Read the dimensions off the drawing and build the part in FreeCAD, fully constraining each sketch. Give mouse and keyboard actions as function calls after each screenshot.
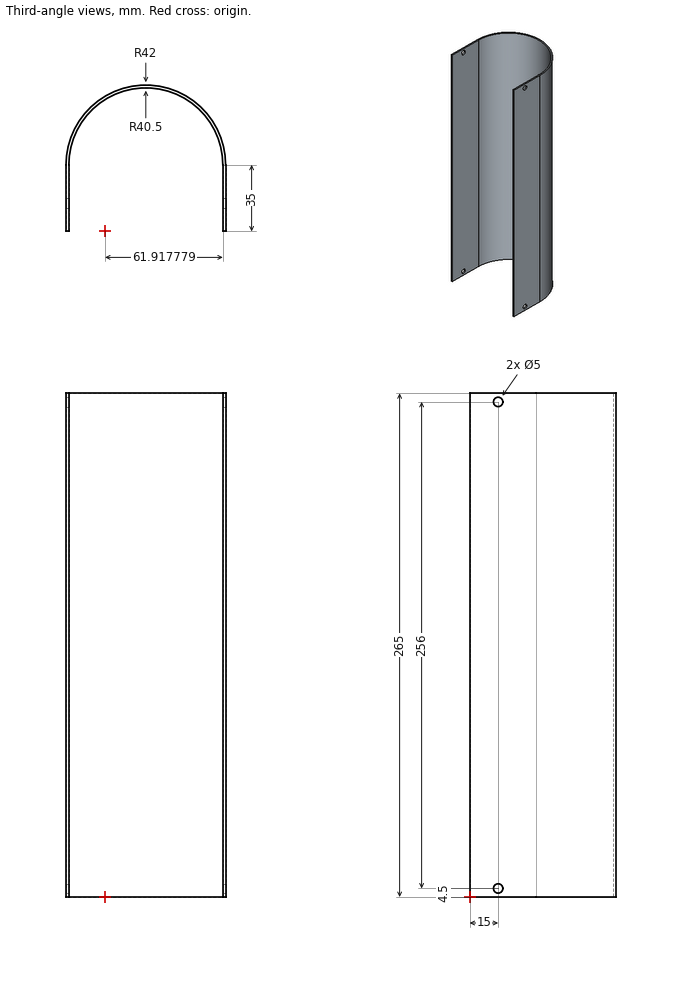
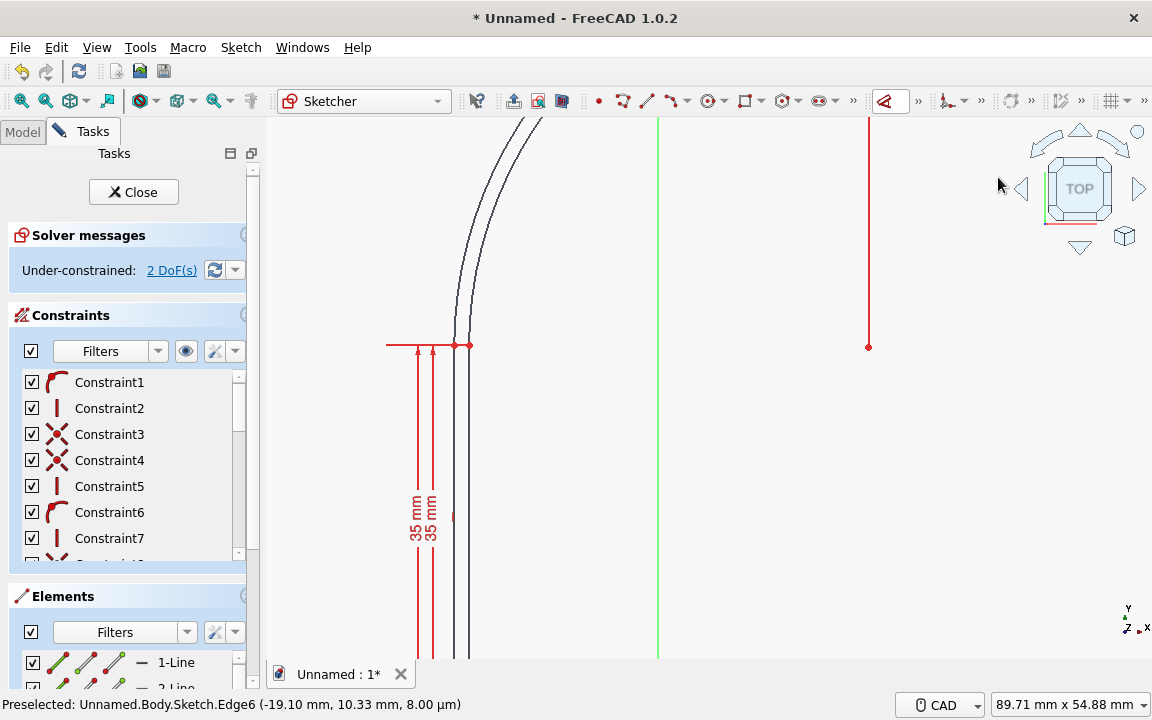
click(869, 347)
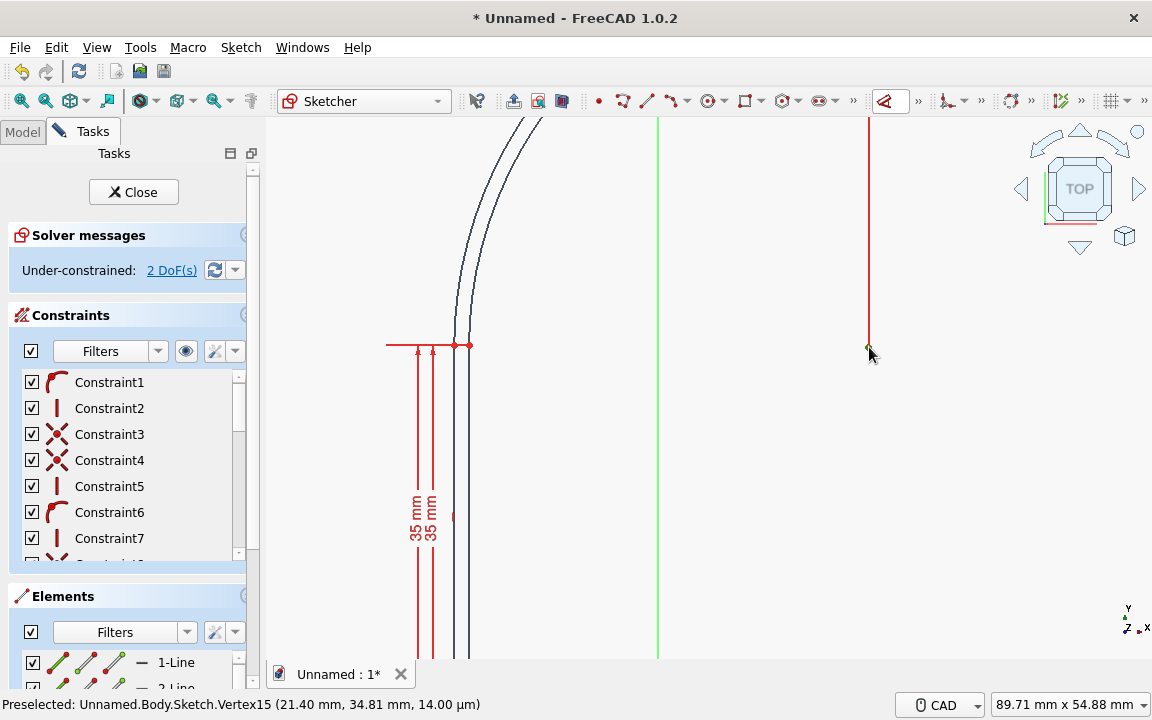
key(i)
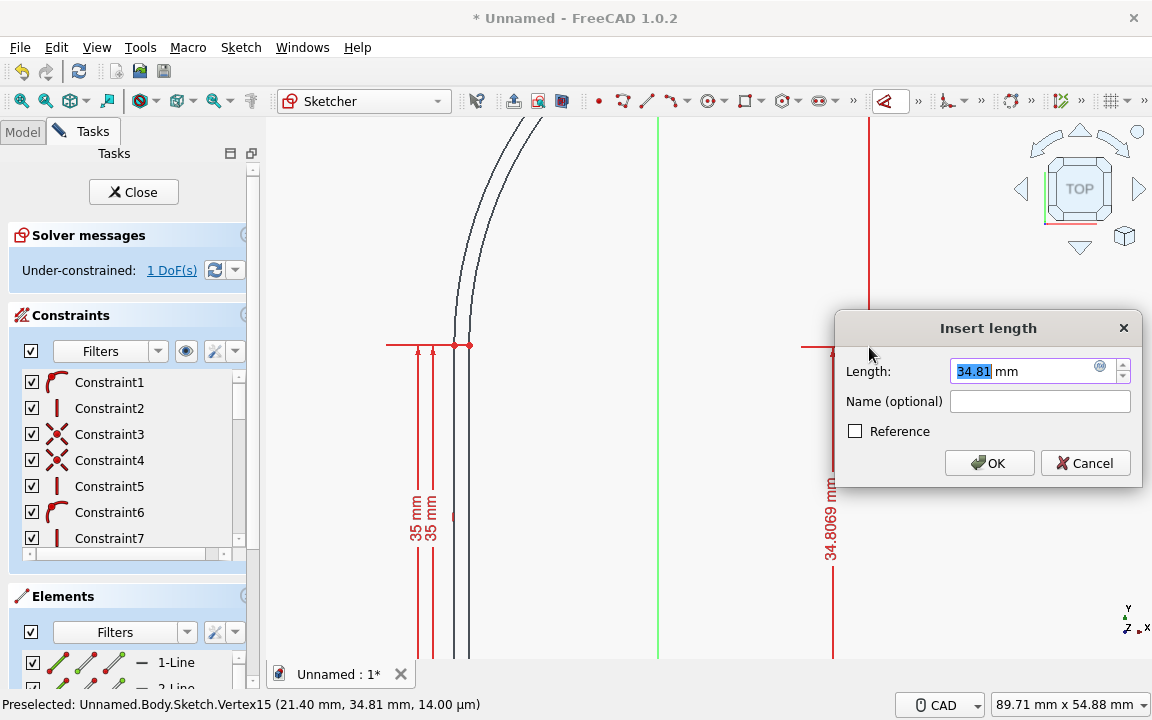
text(35)
key(Return)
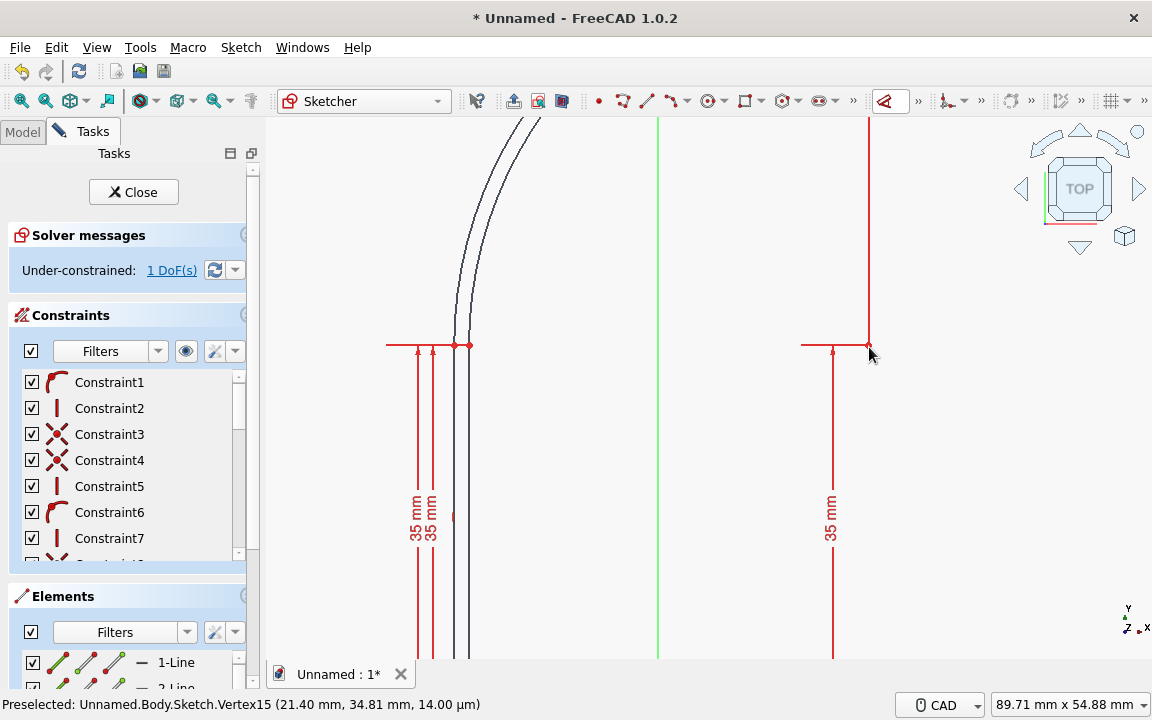
scroll(454, 451, down, 4)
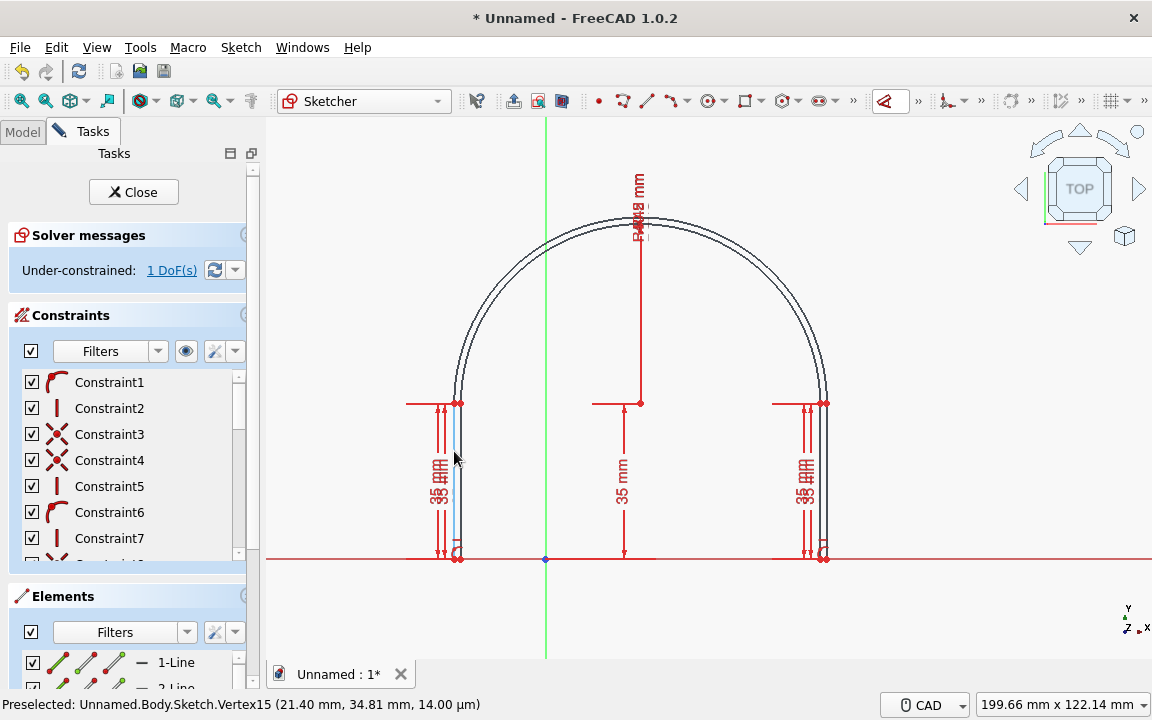
scroll(820, 404, up, 4)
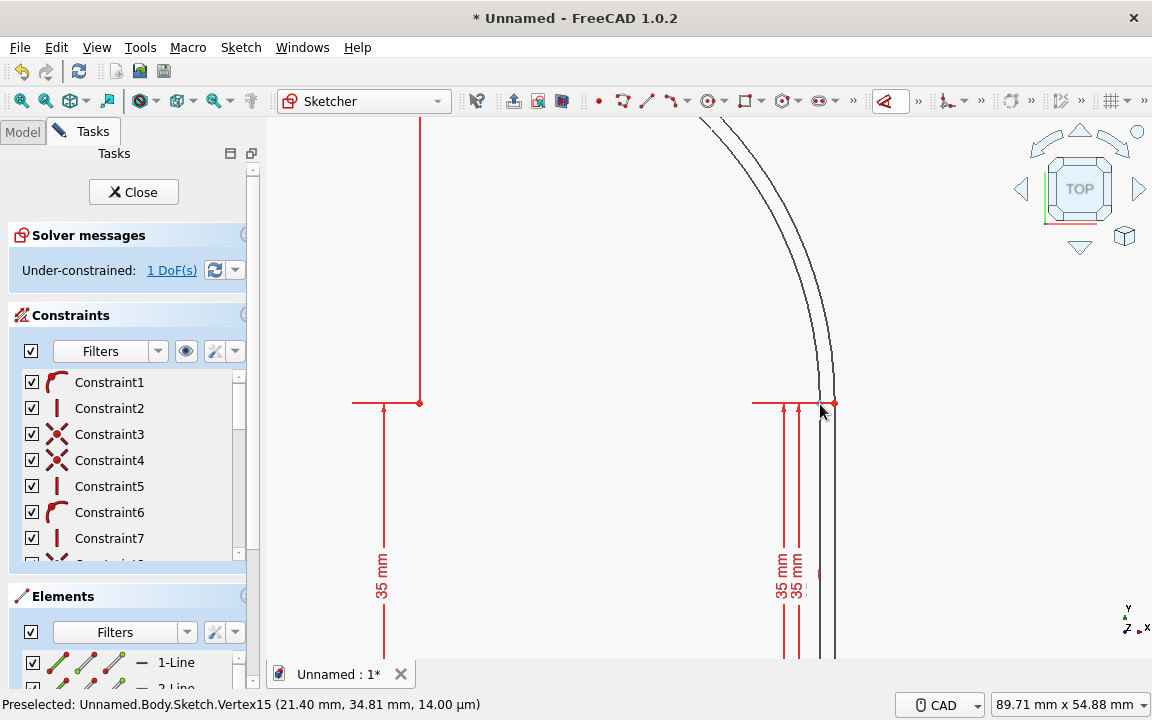
click(820, 403)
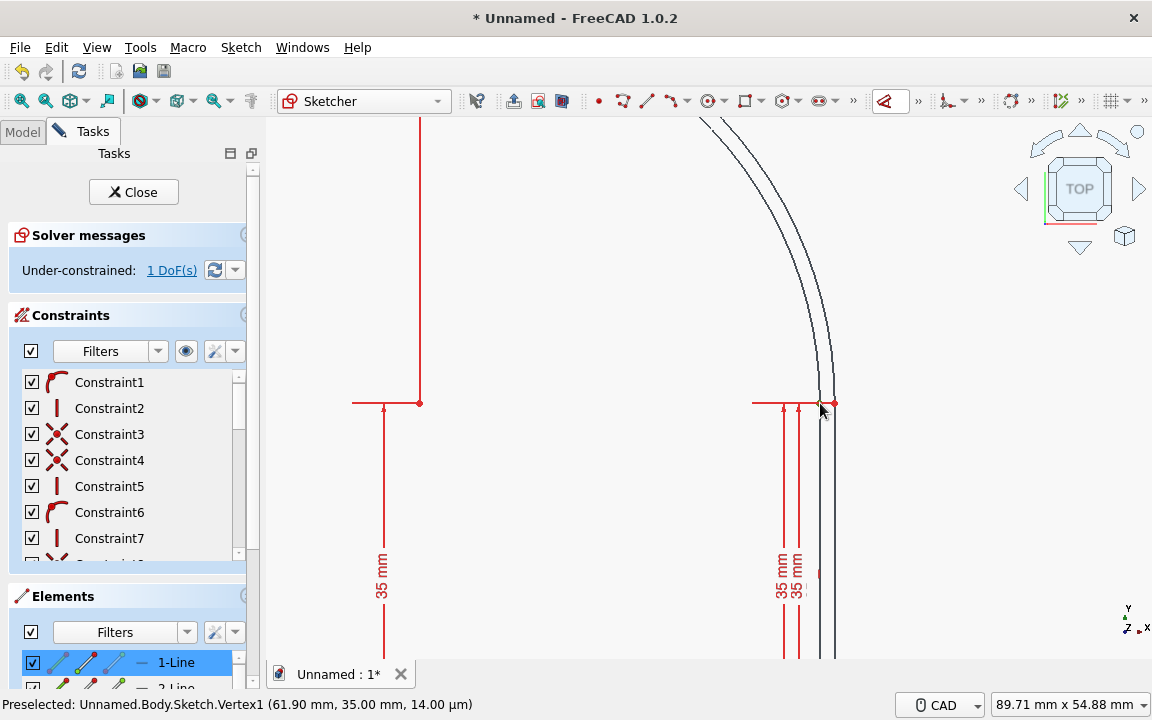
click(904, 102)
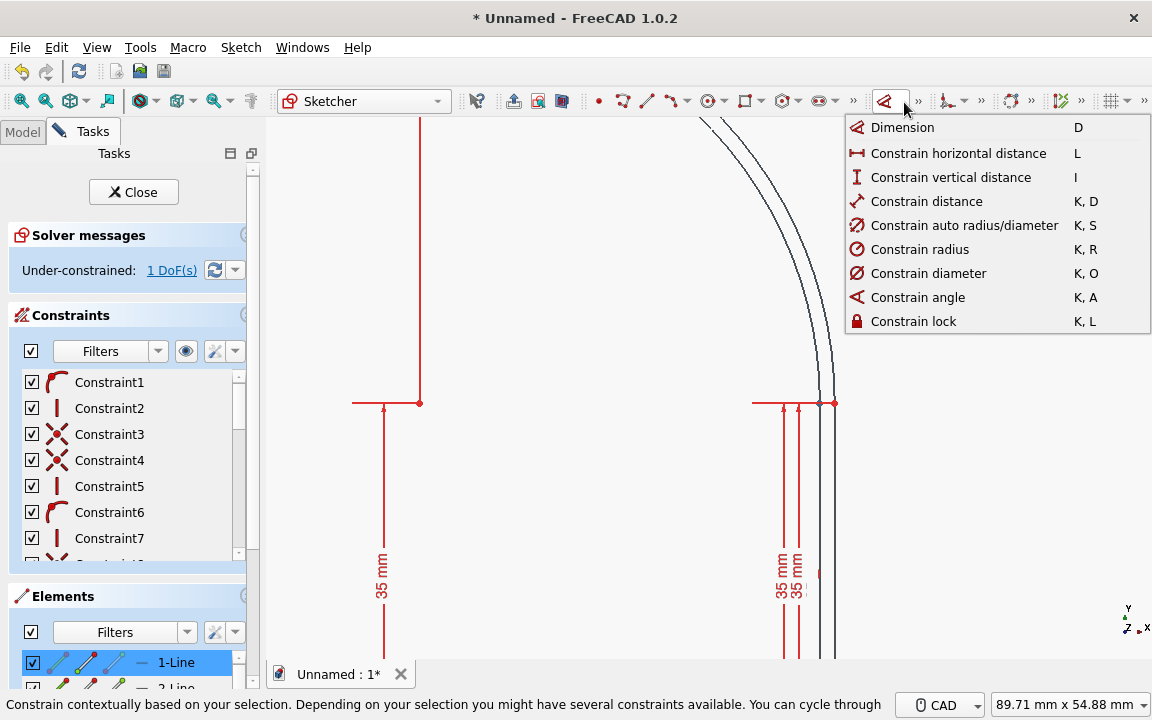
click(998, 153)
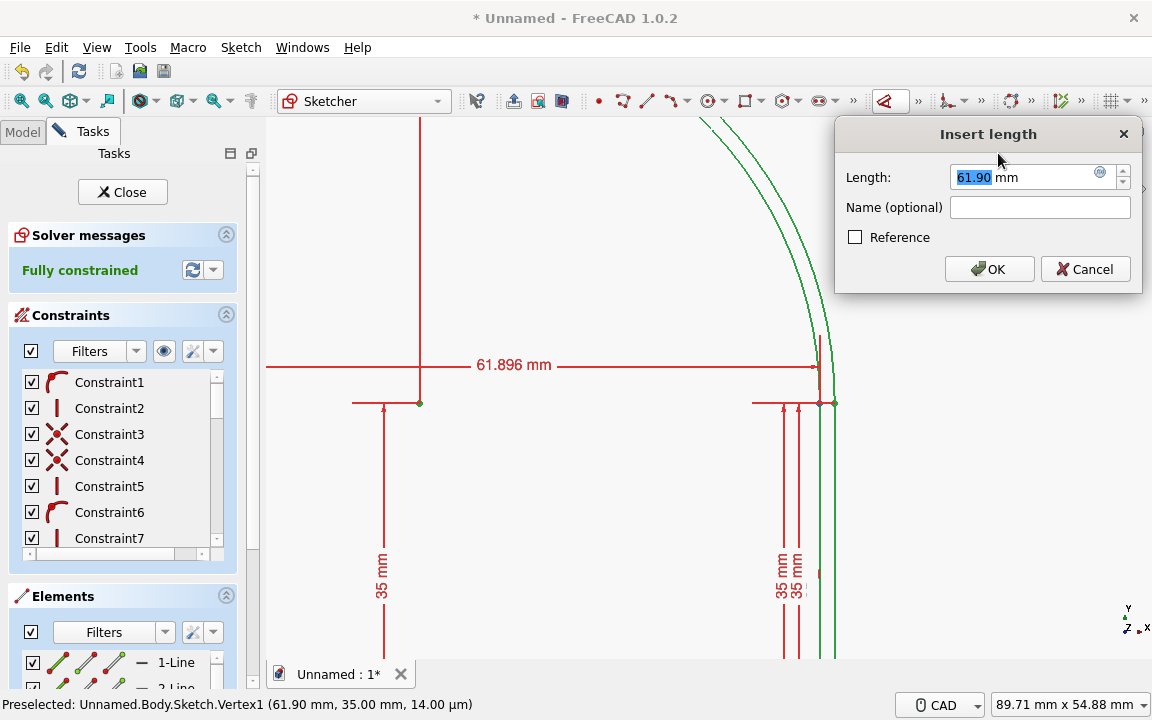
text(61.917779)
key(Return)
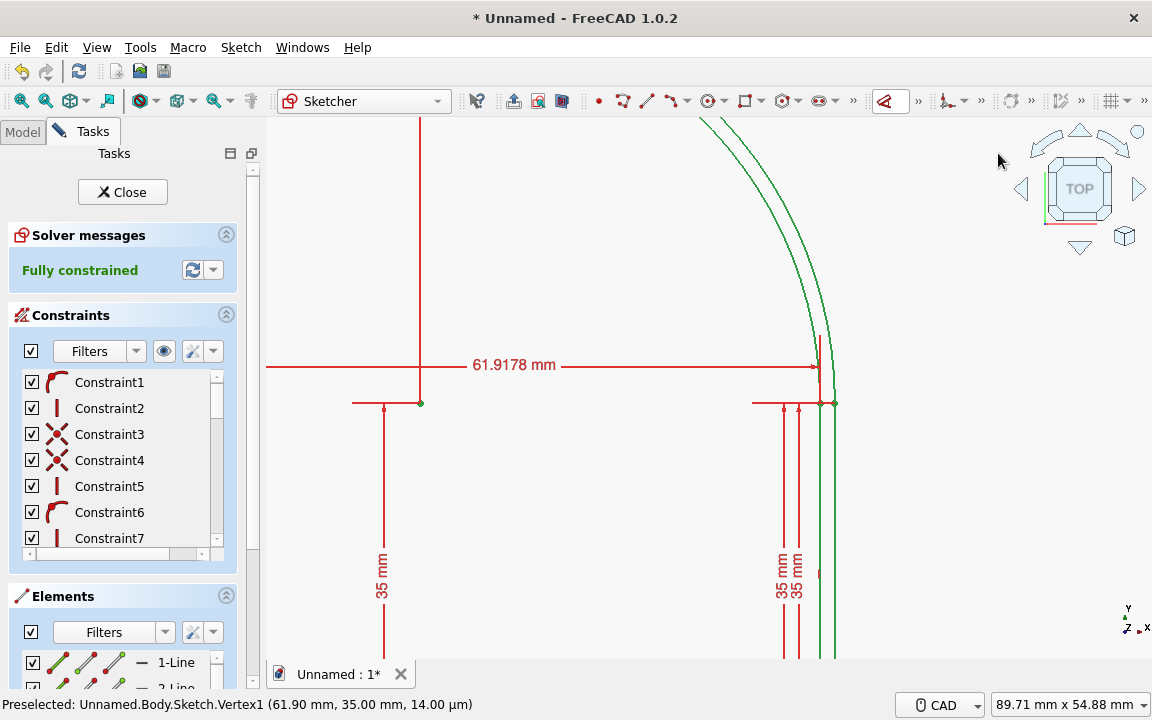
click(123, 192)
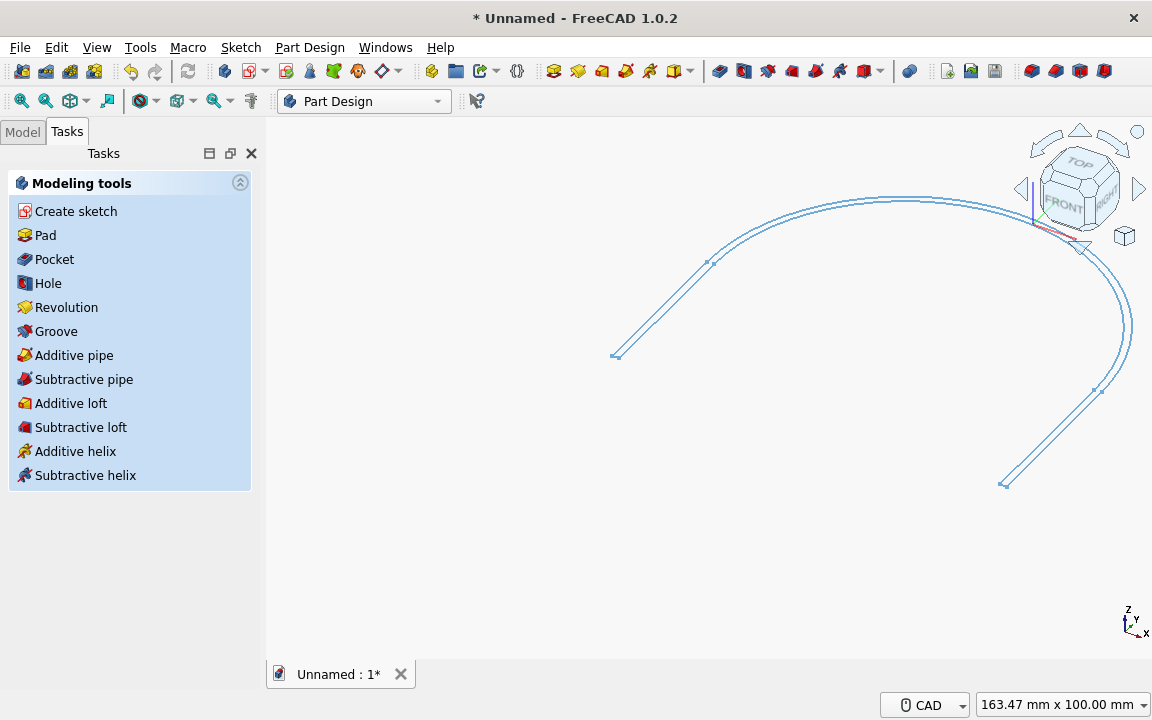
click(554, 72)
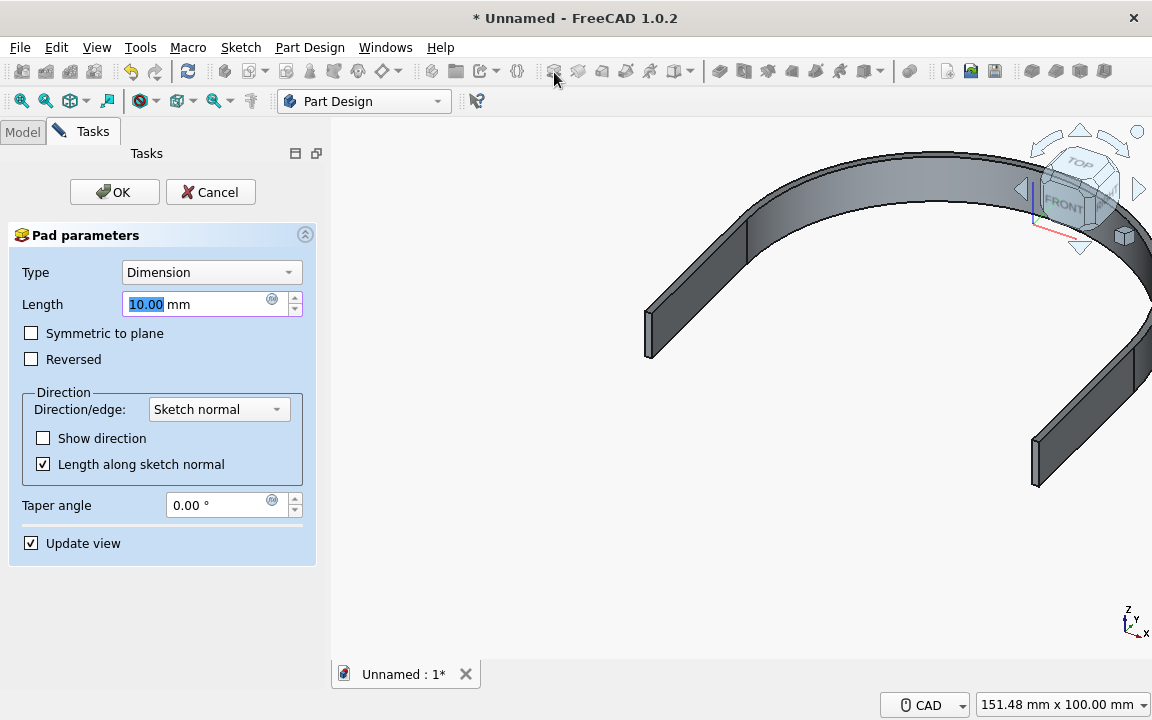
text(265)
key(Tab)